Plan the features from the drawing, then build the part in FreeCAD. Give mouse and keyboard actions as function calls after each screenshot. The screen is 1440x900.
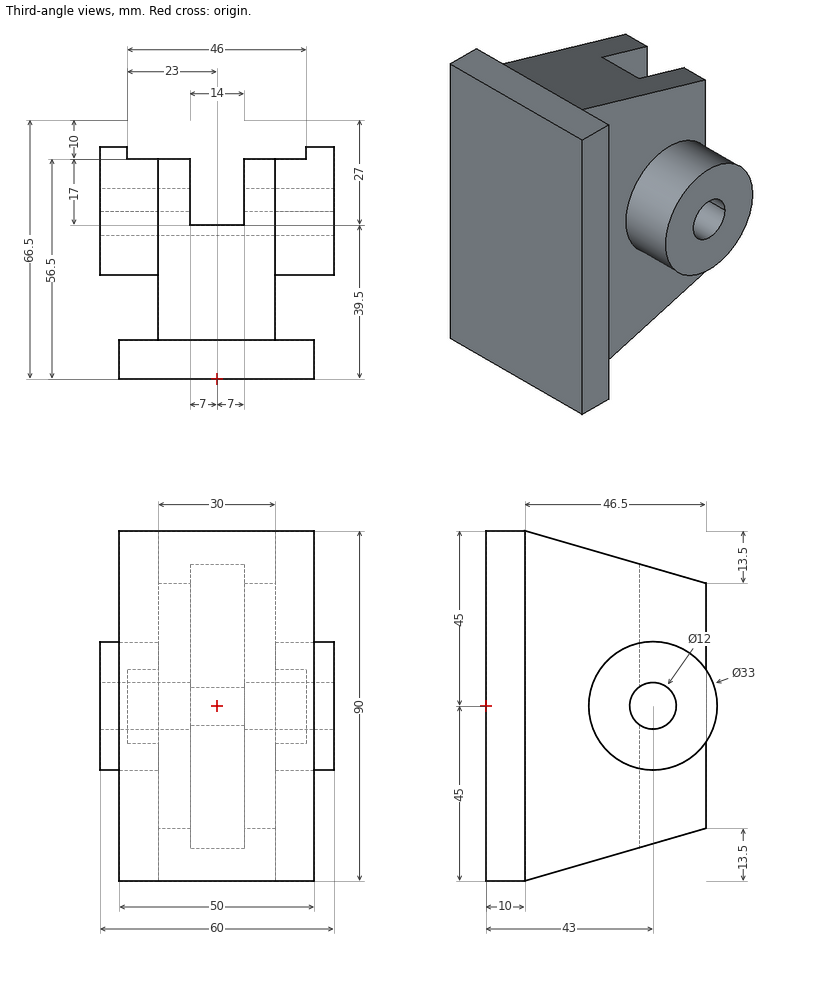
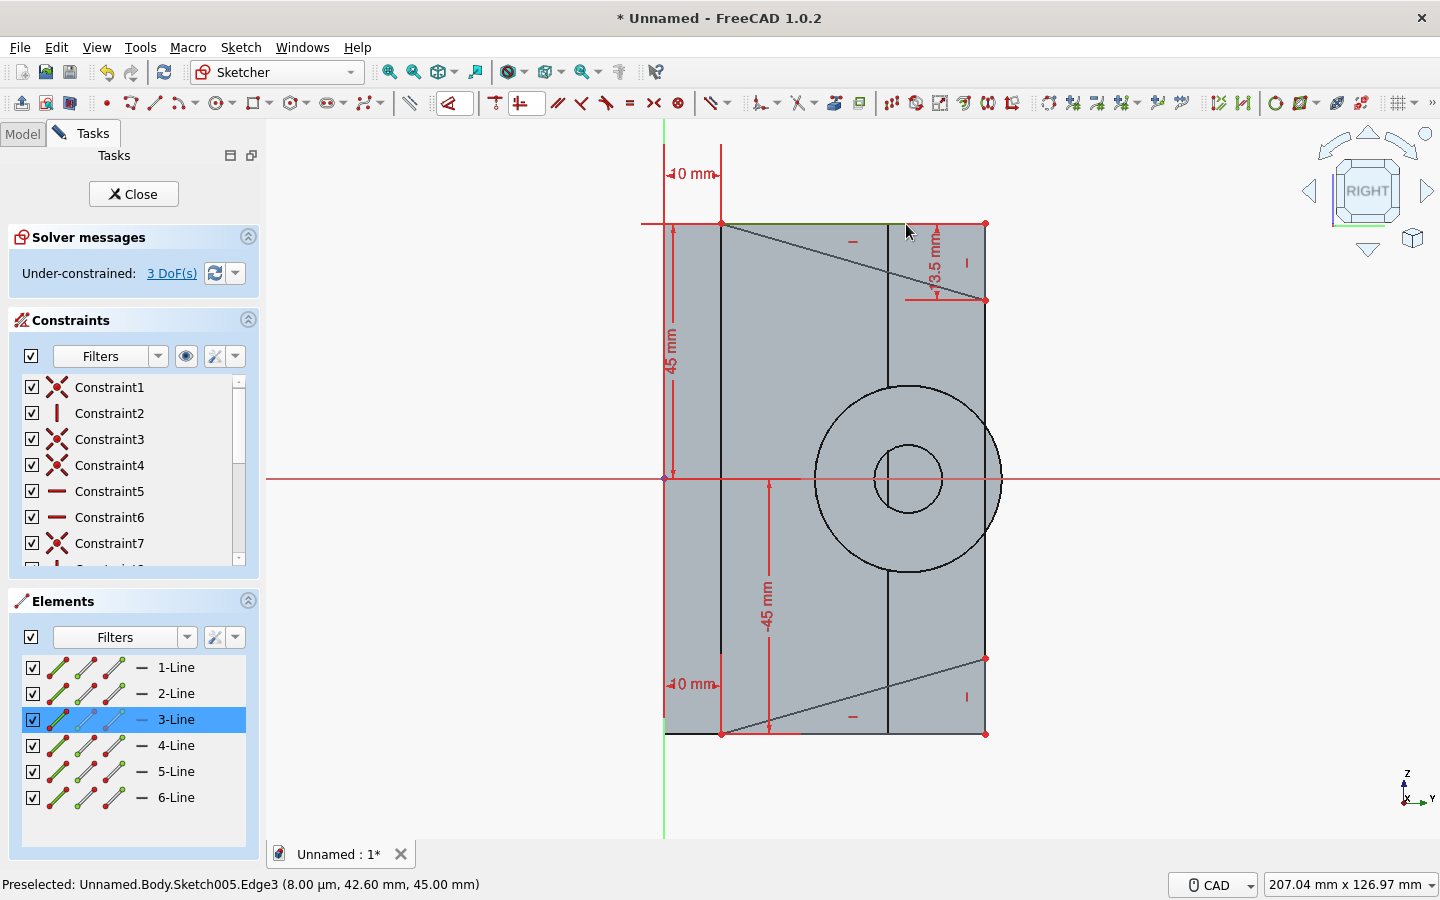
click(468, 104)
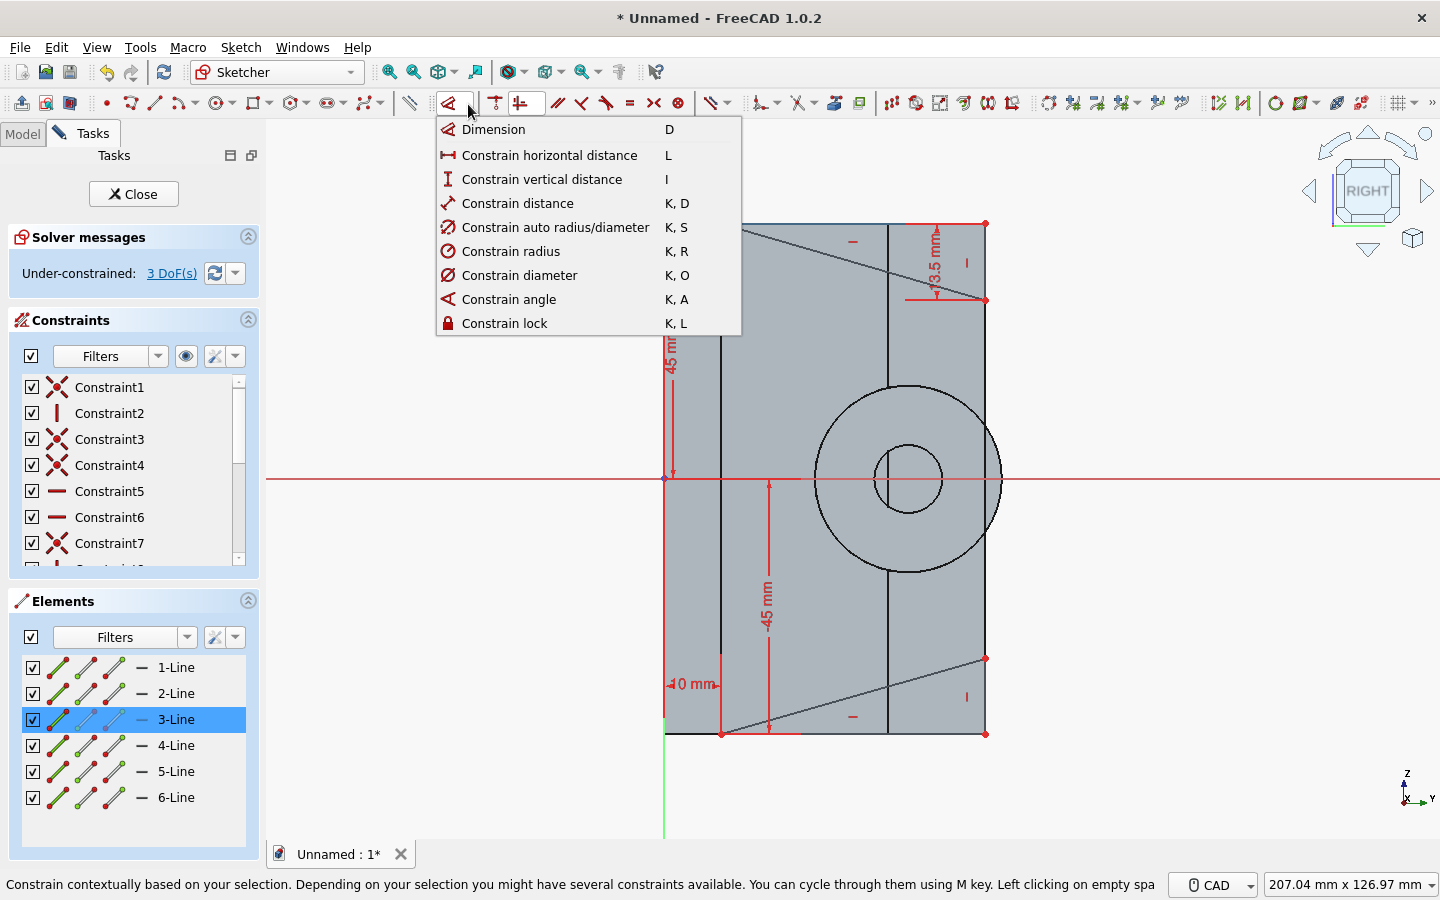
click(589, 155)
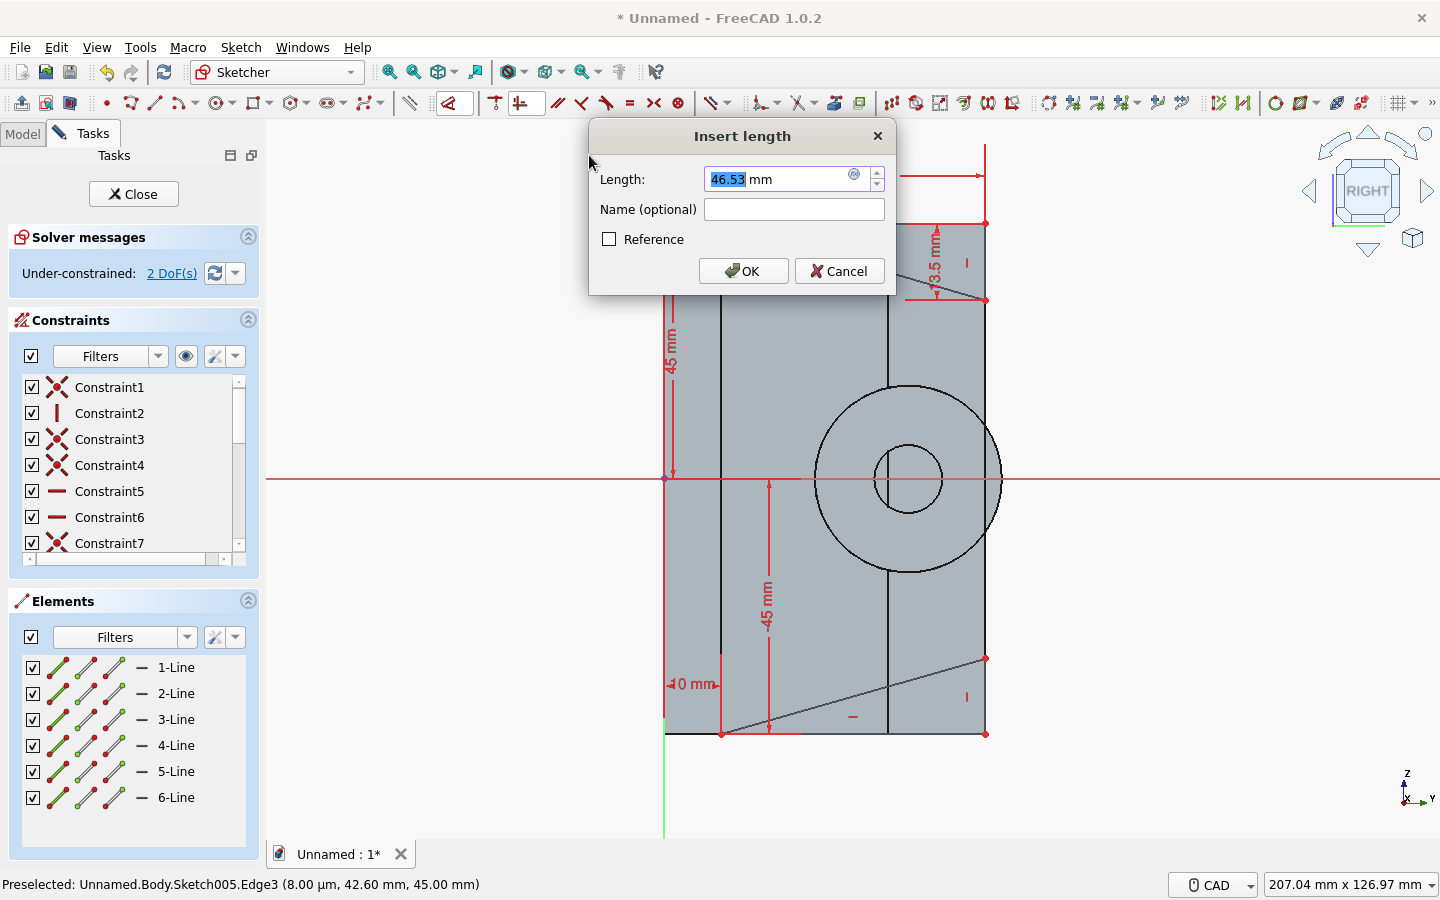
text(46.5)
key(Return)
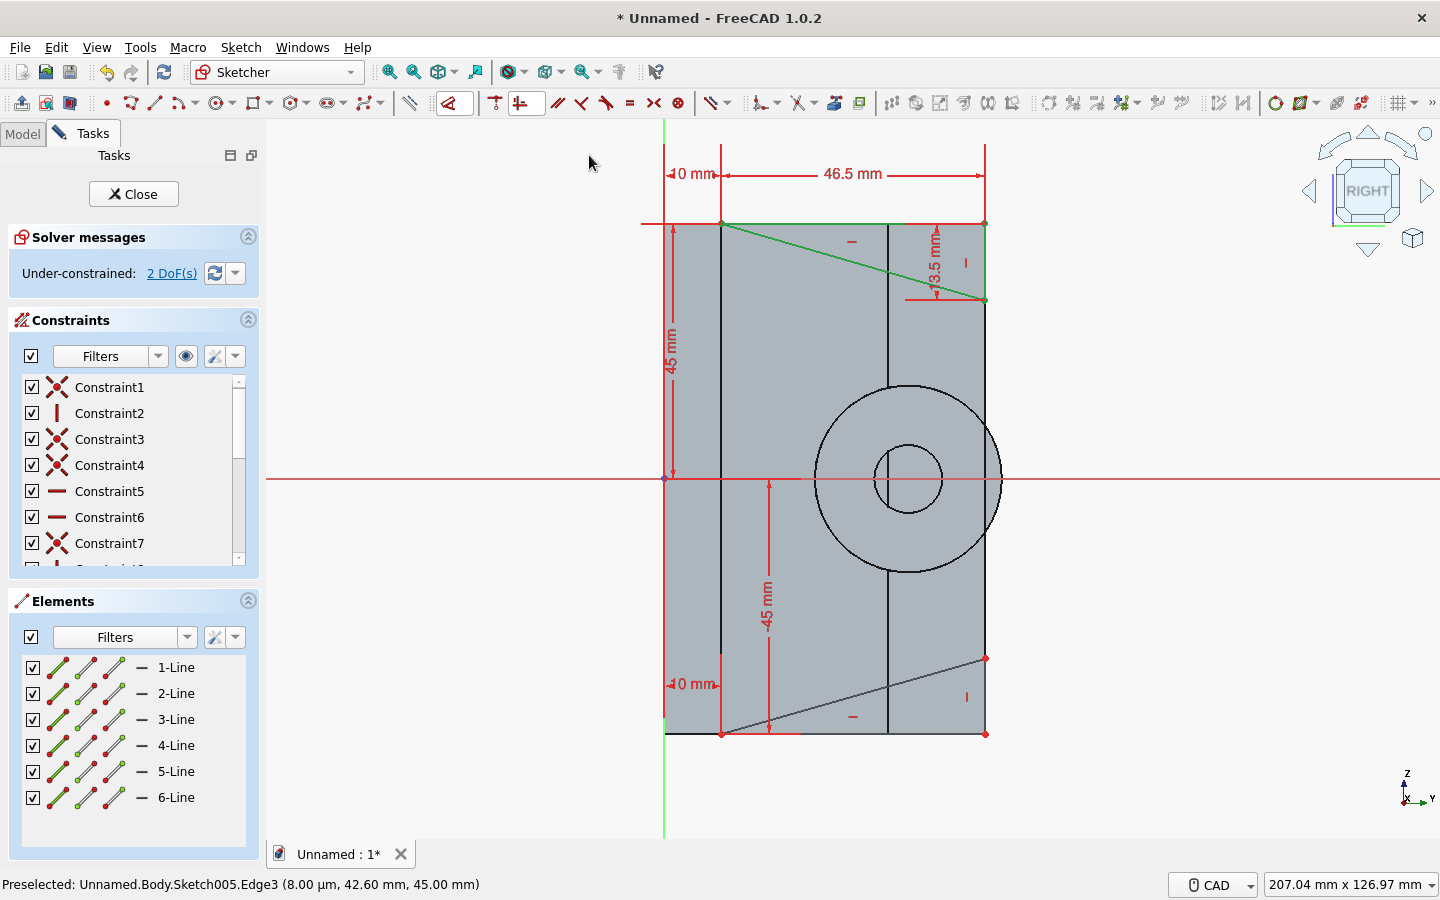
click(800, 734)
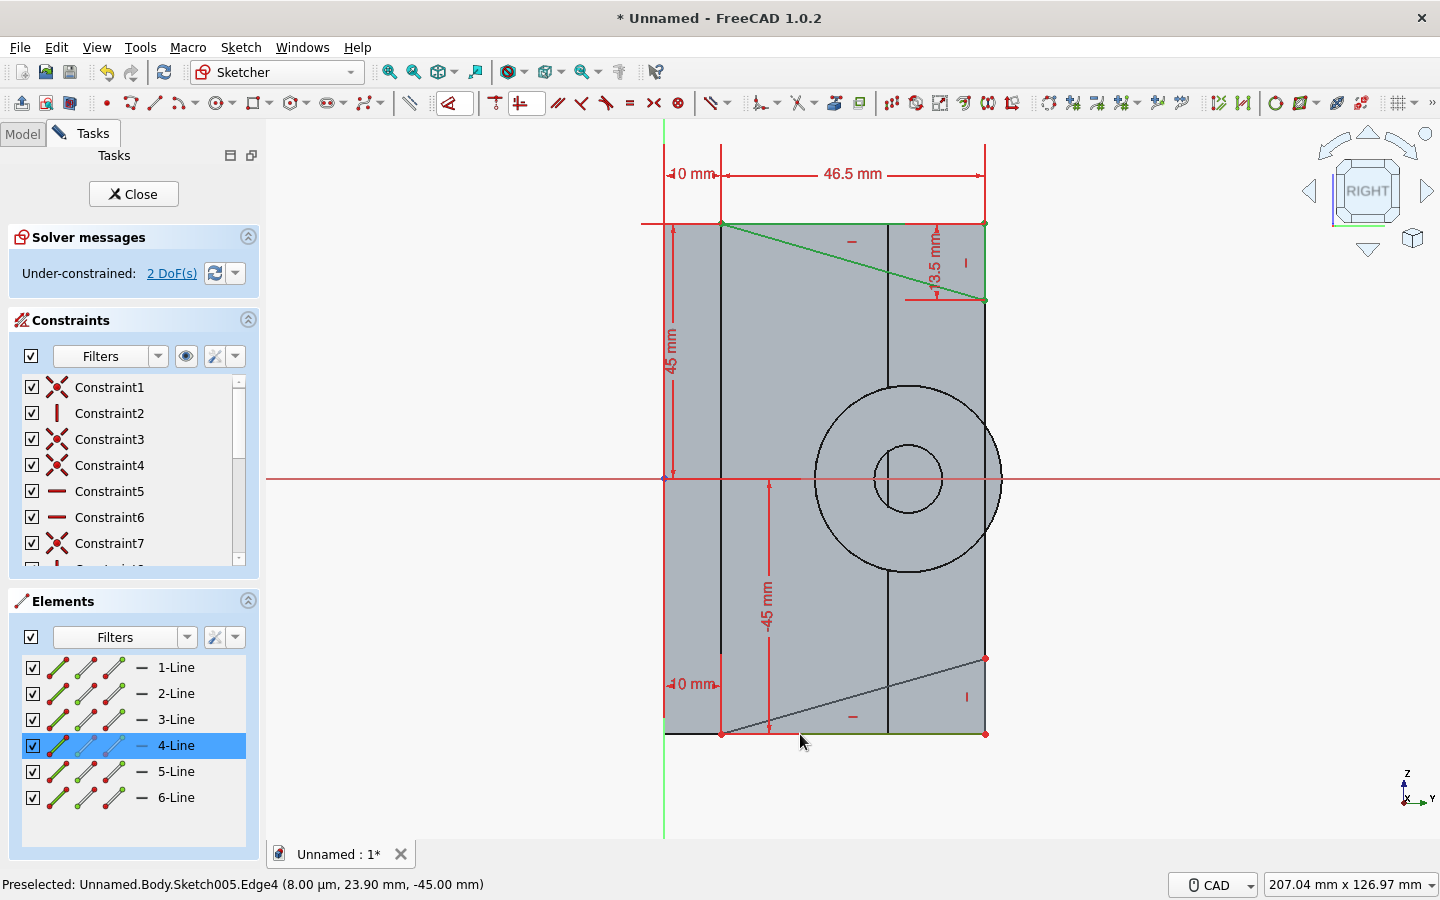
click(468, 104)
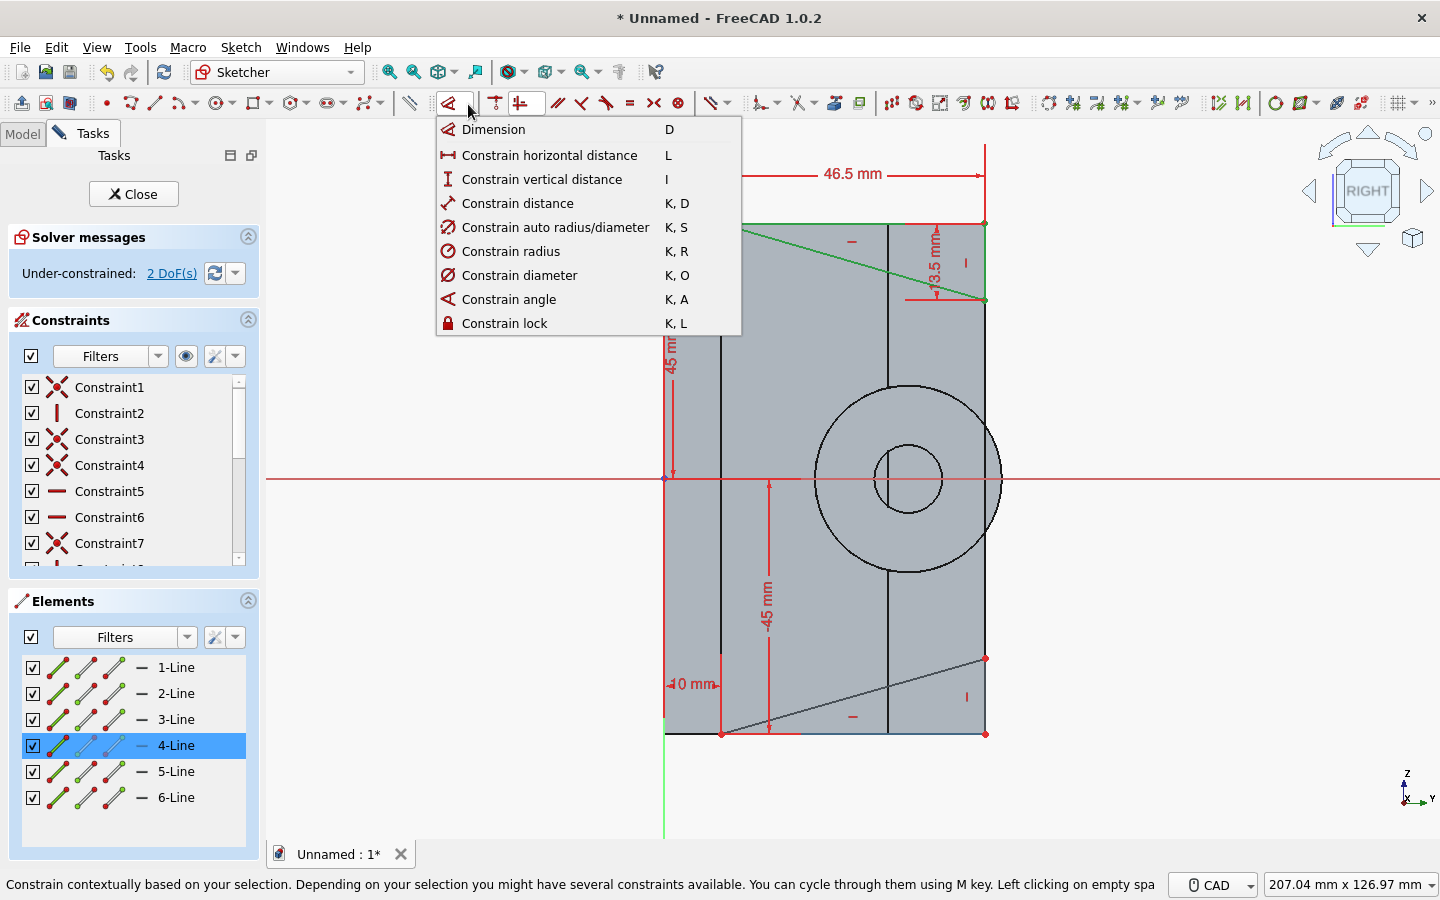
click(589, 155)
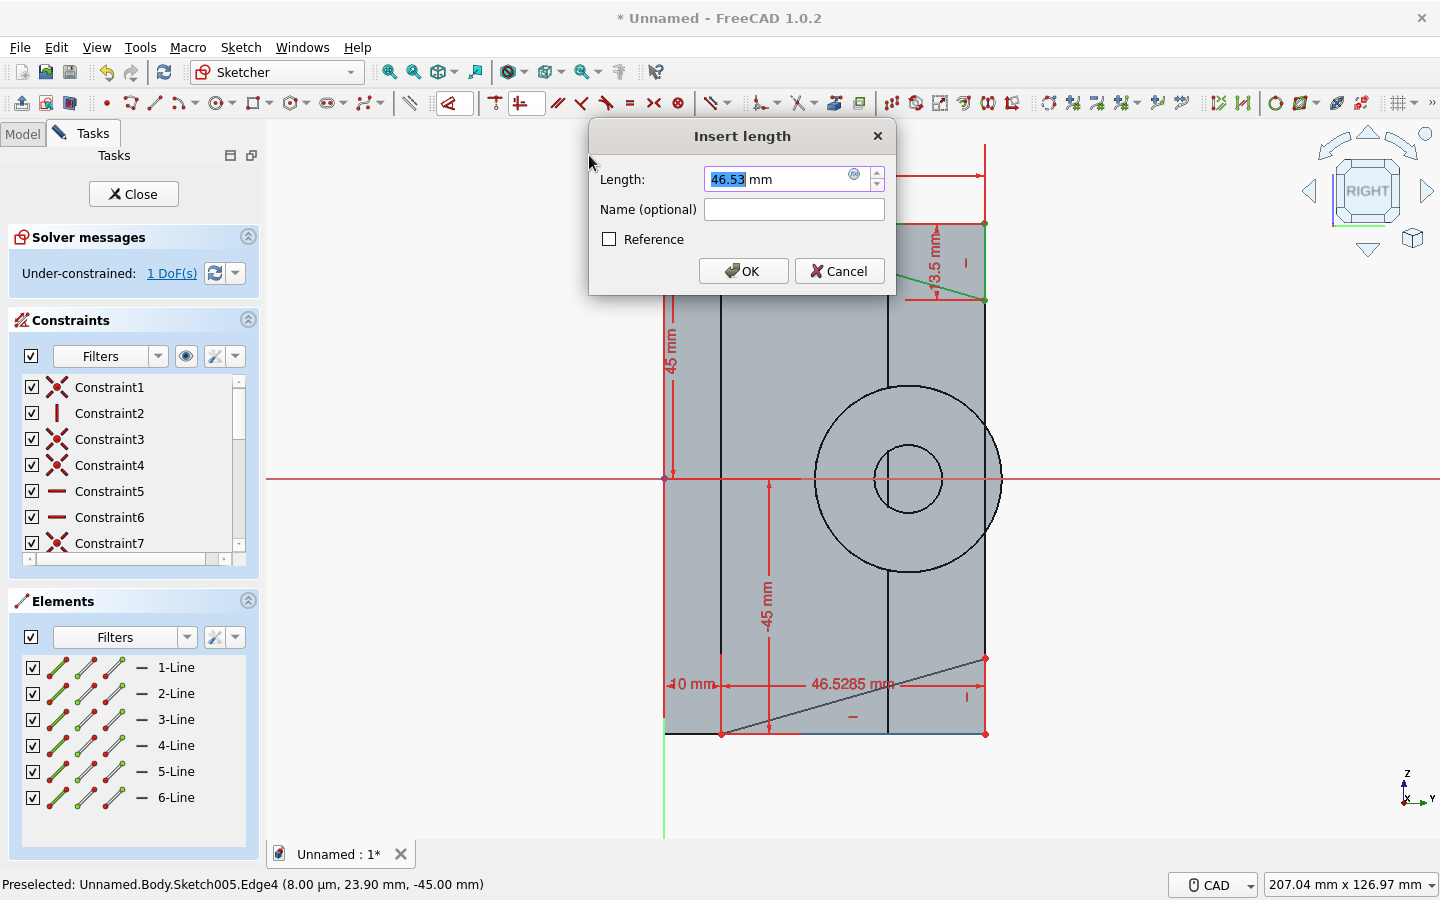
text(46.5)
key(Return)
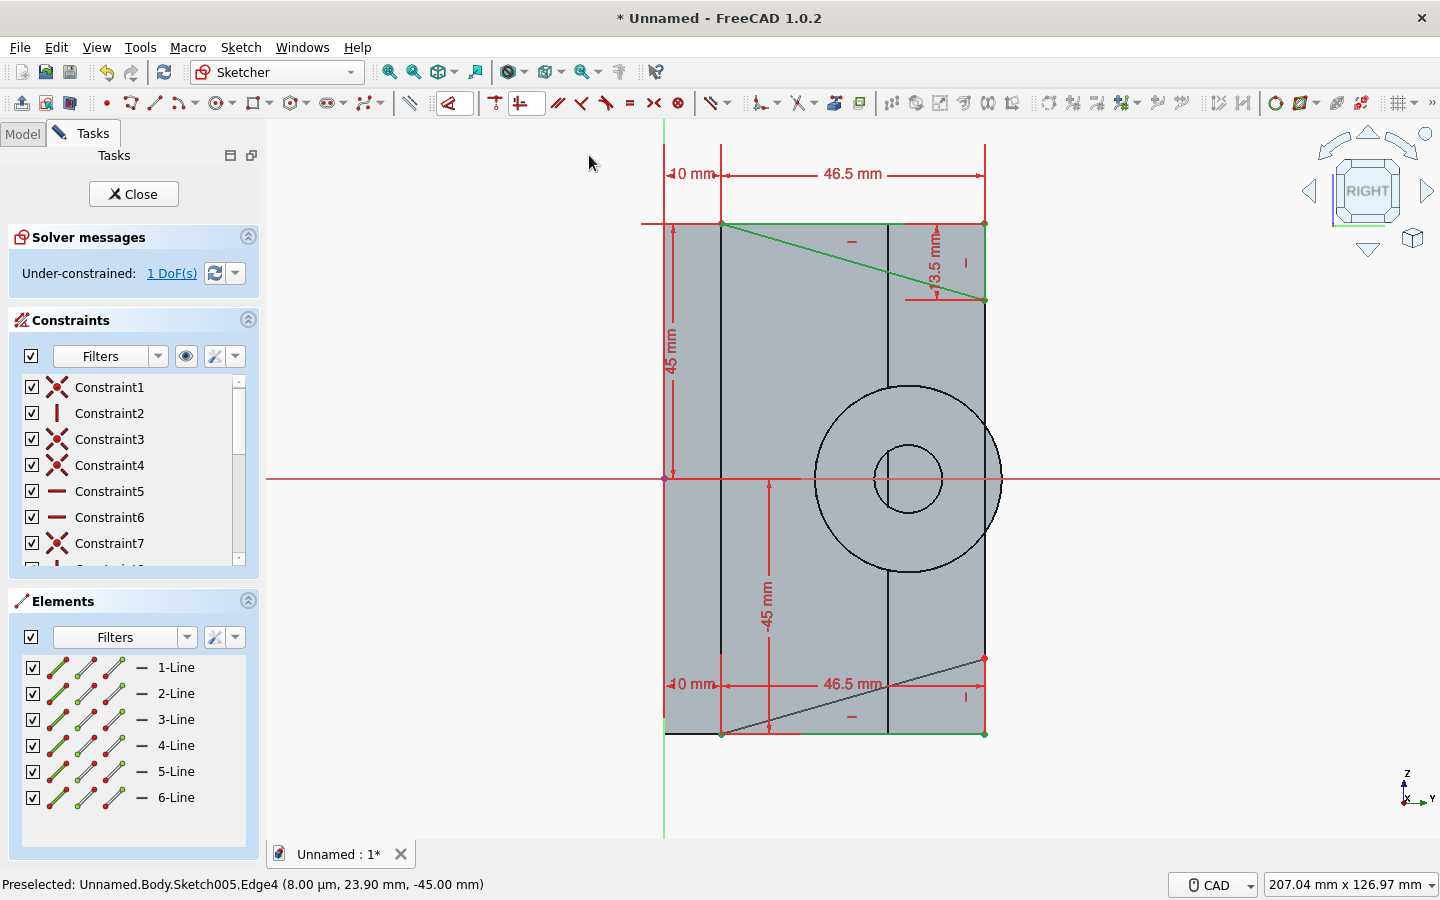
click(985, 712)